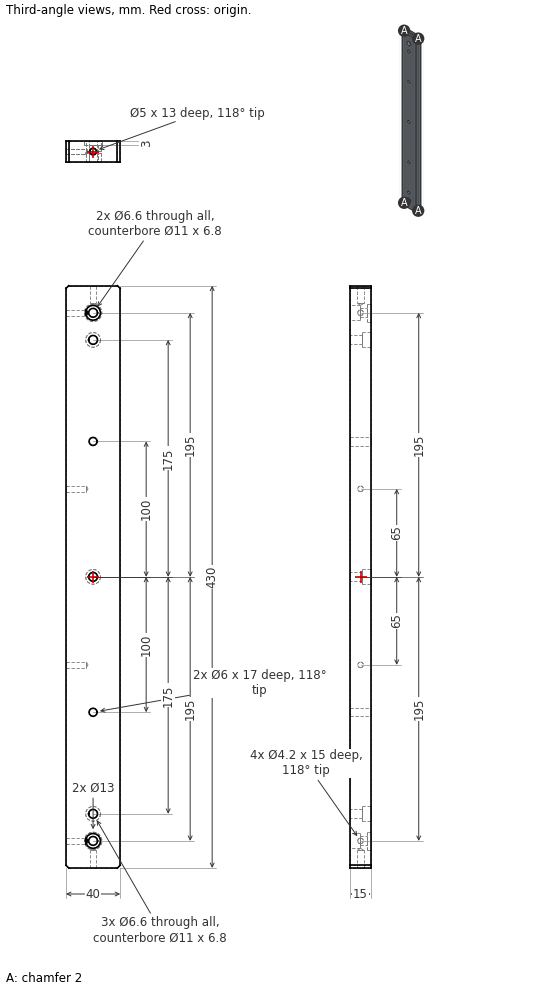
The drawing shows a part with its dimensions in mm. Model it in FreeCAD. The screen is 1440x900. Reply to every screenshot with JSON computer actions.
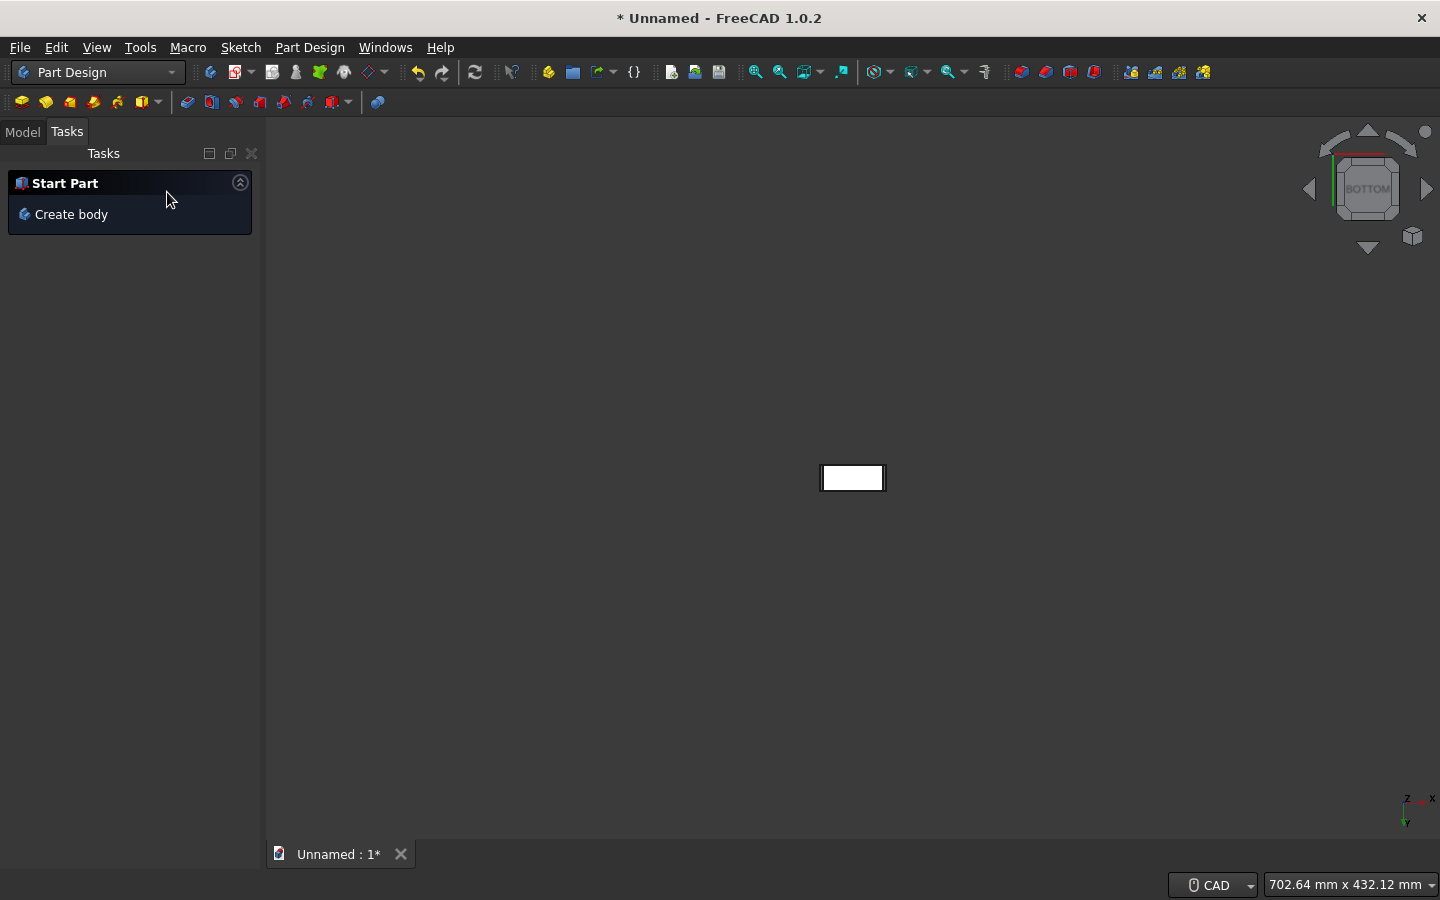
{"action": "left_click", "coordinate": [870, 477]}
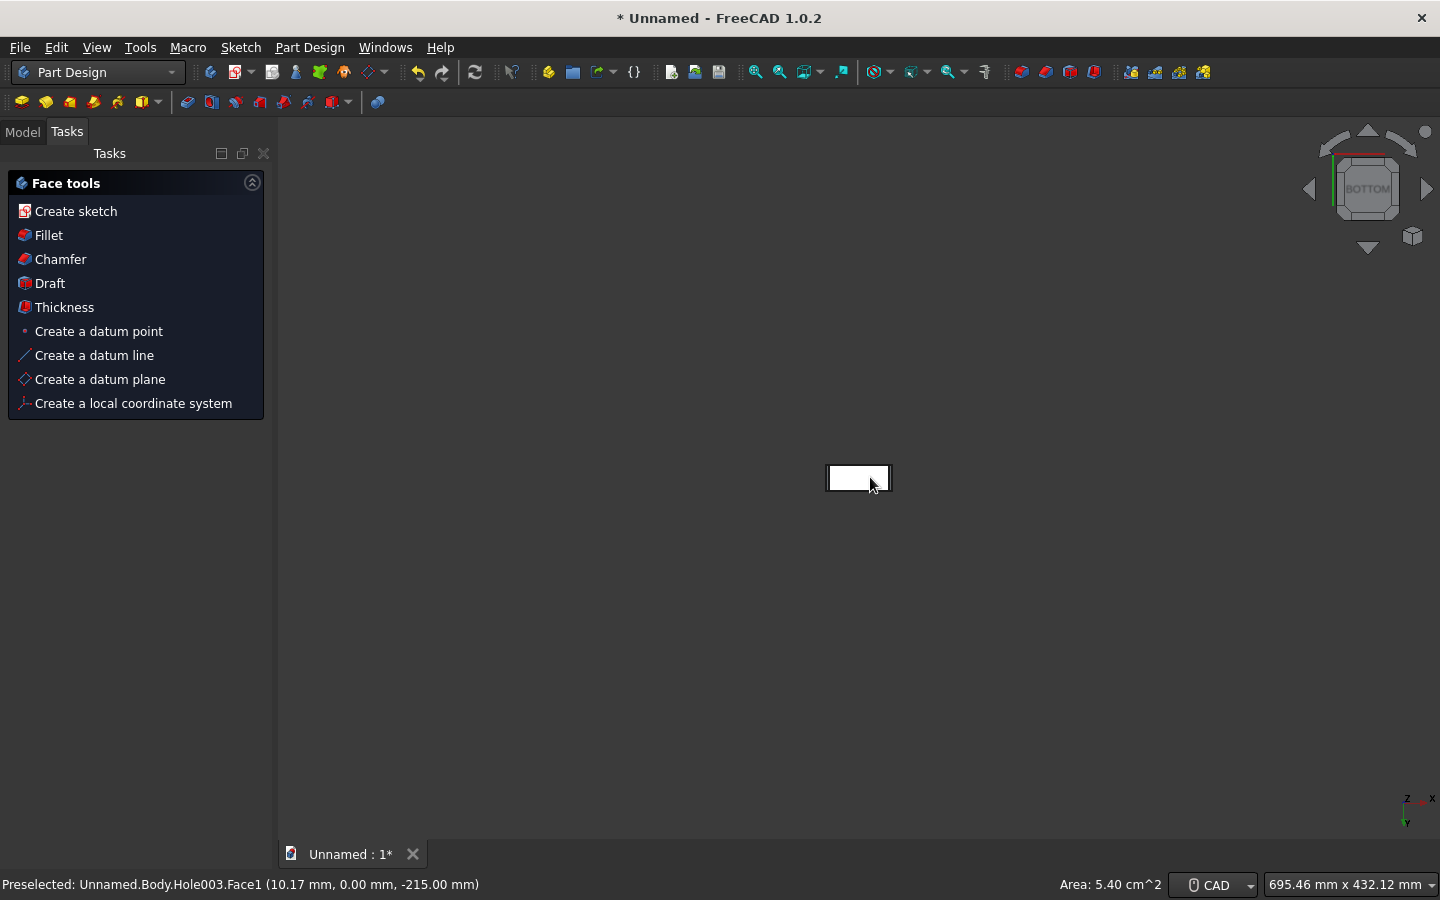
{"action": "left_click", "coordinate": [236, 72]}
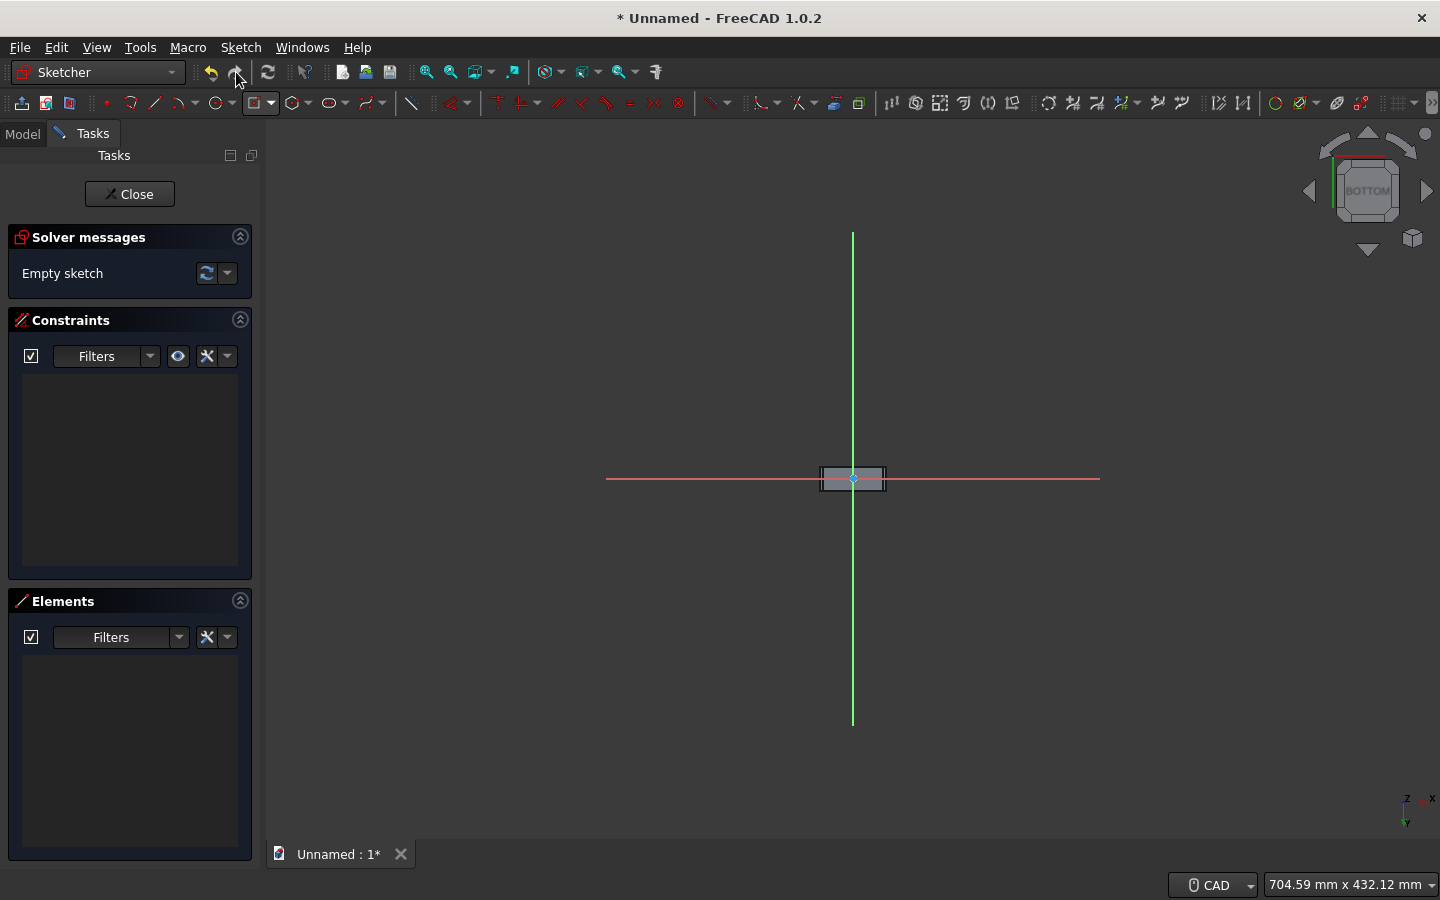
{"action": "scroll", "coordinate": [857, 479], "scroll_direction": "up", "scroll_amount": 15}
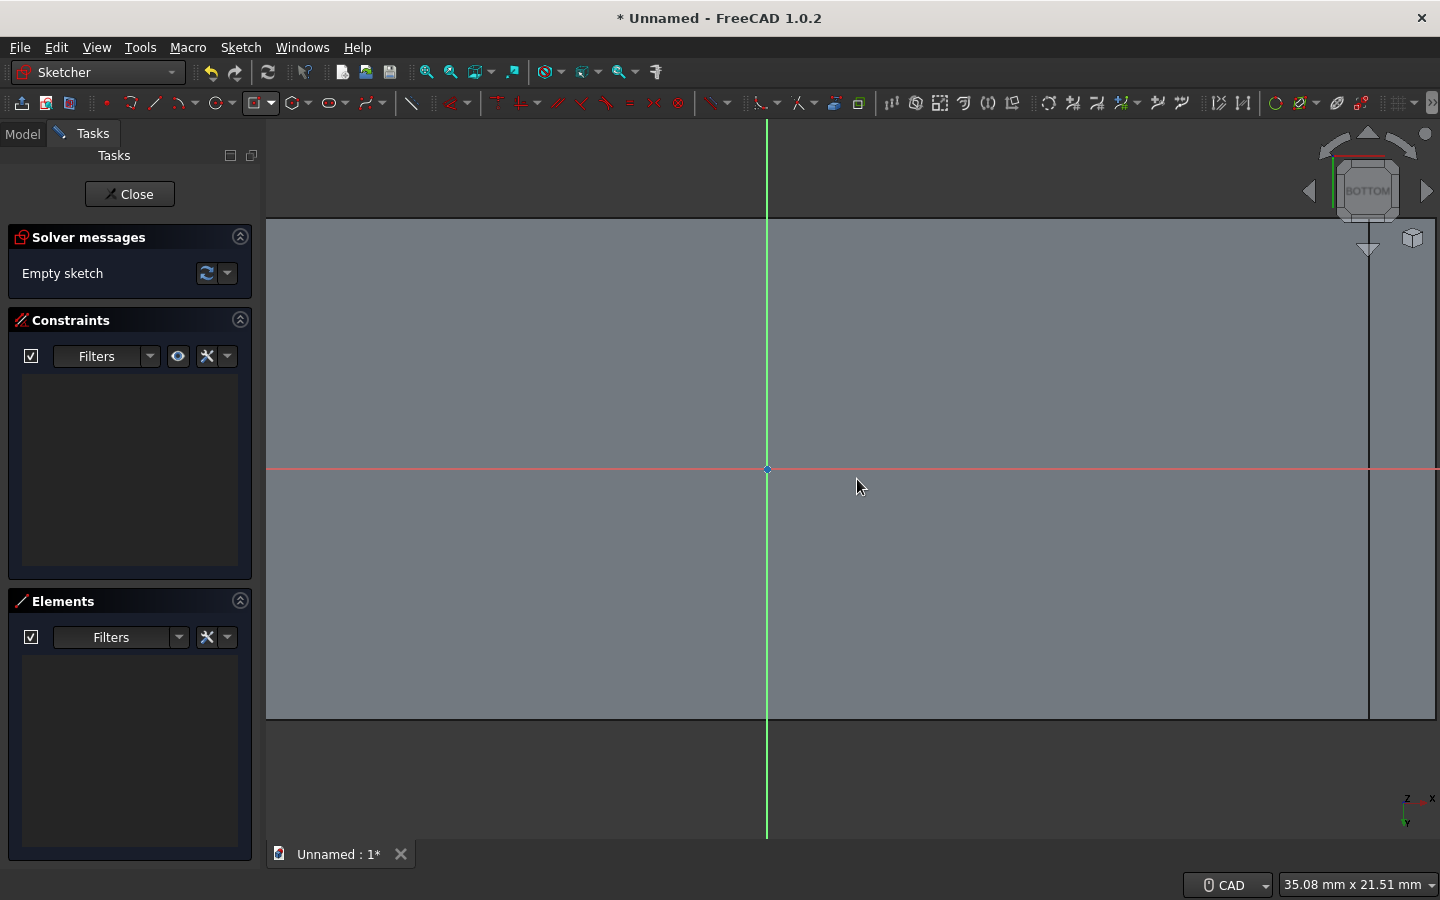
{"action": "scroll", "coordinate": [757, 464], "scroll_direction": "up", "scroll_amount": 5}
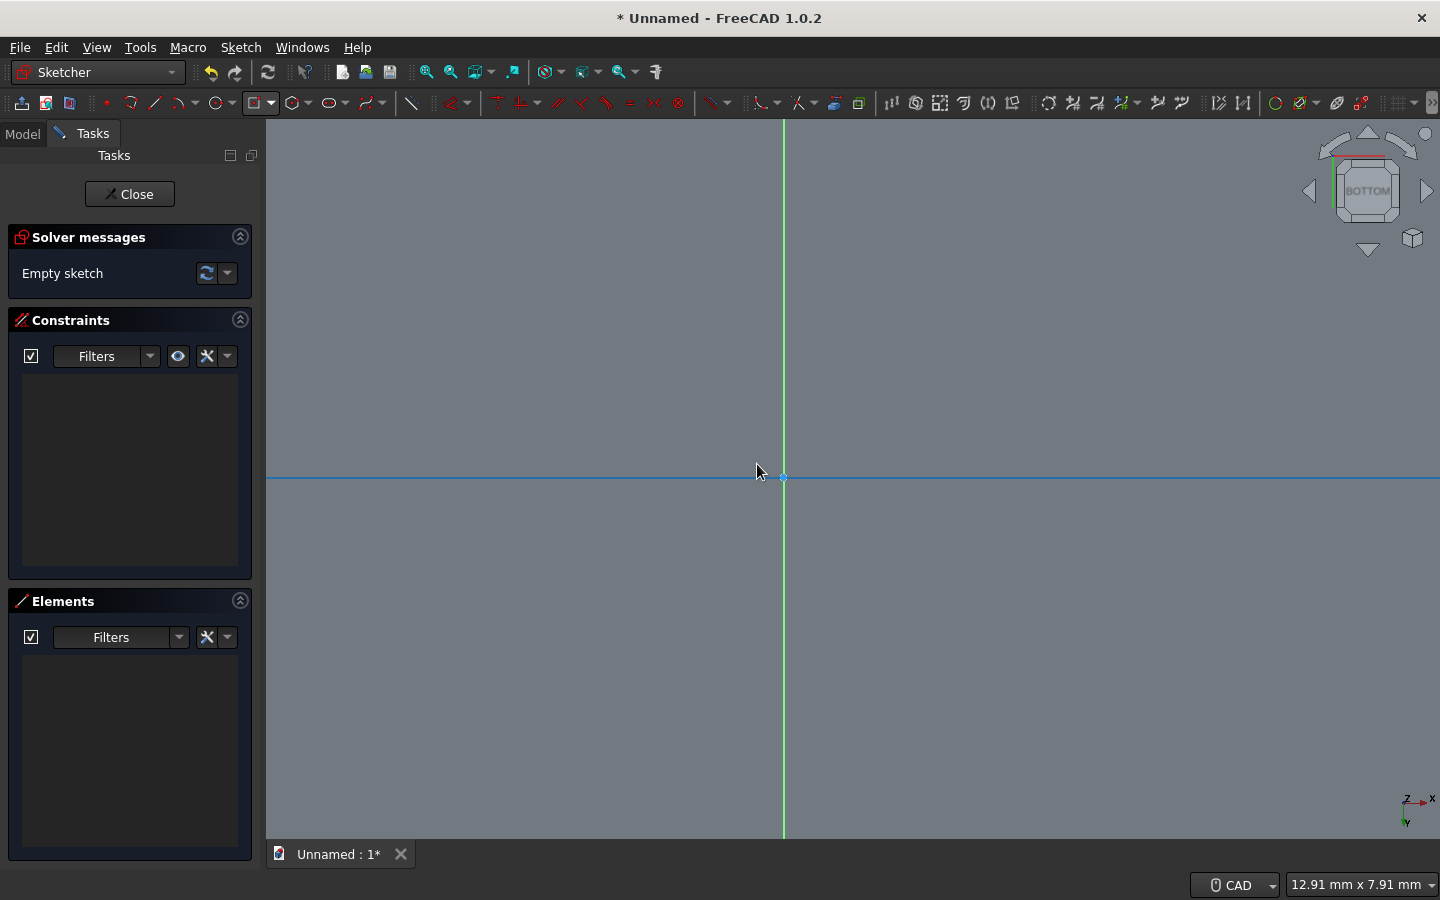
{"action": "key", "text": "g c"}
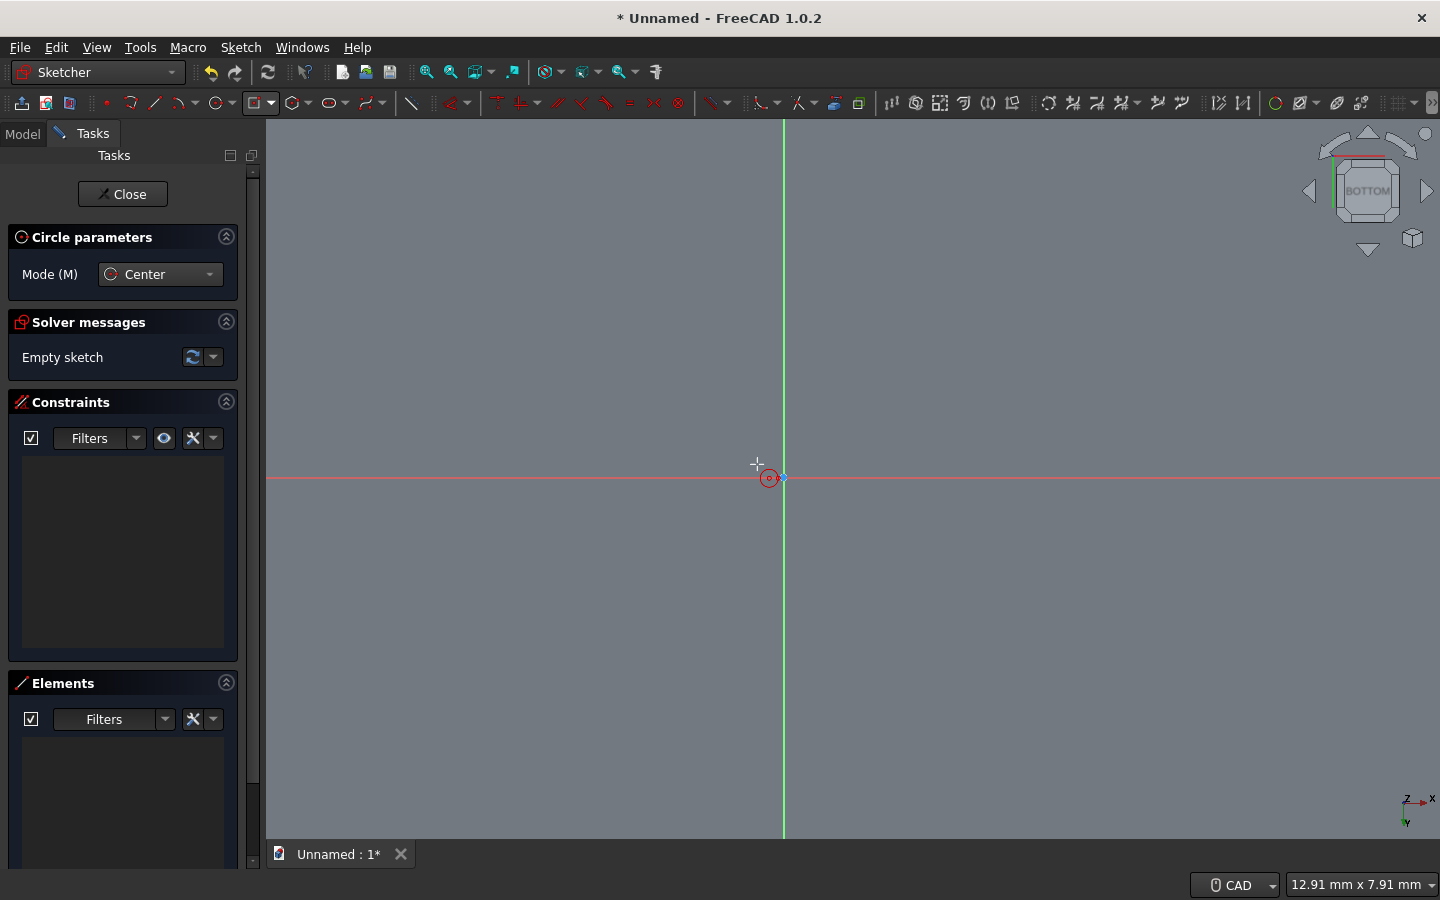
{"action": "left_click", "coordinate": [784, 478]}
{"action": "left_click", "coordinate": [944, 317]}
{"action": "key", "text": "Escape"}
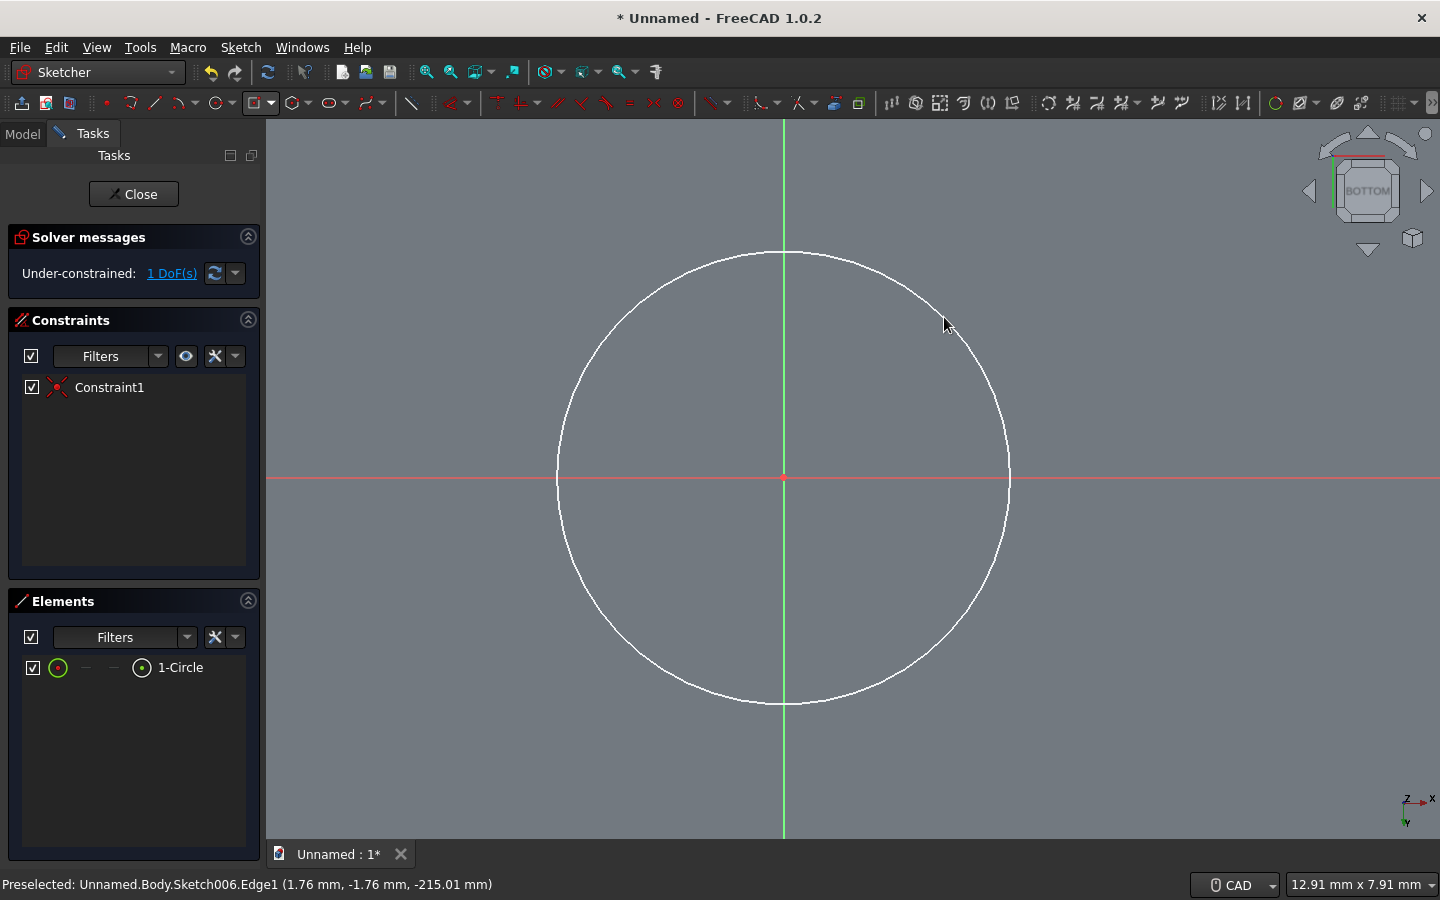
{"action": "key", "text": "d"}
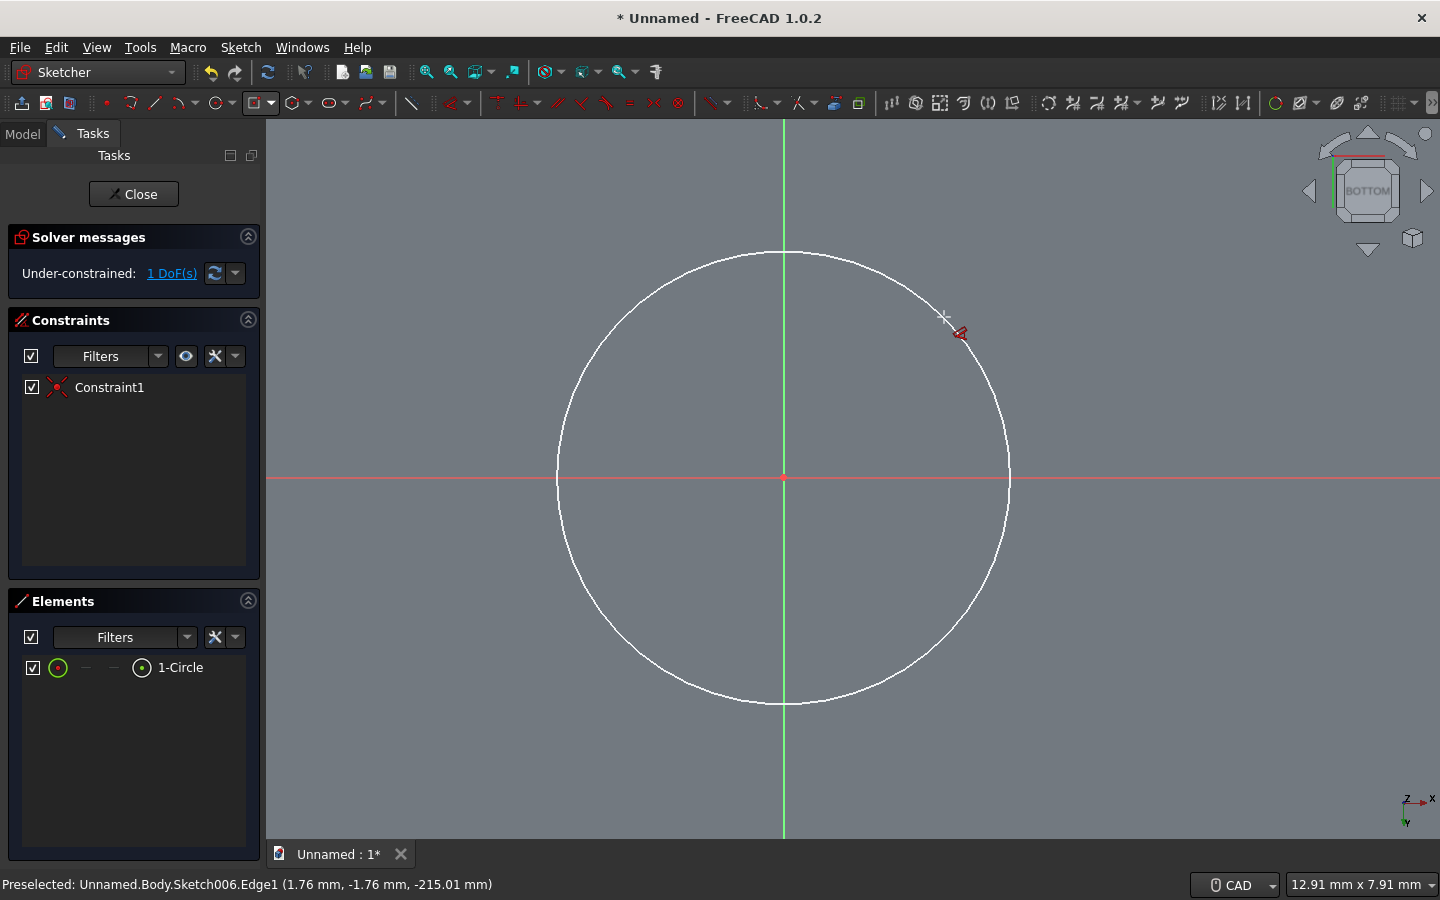
{"action": "left_click", "coordinate": [943, 317]}
{"action": "left_click", "coordinate": [966, 294]}